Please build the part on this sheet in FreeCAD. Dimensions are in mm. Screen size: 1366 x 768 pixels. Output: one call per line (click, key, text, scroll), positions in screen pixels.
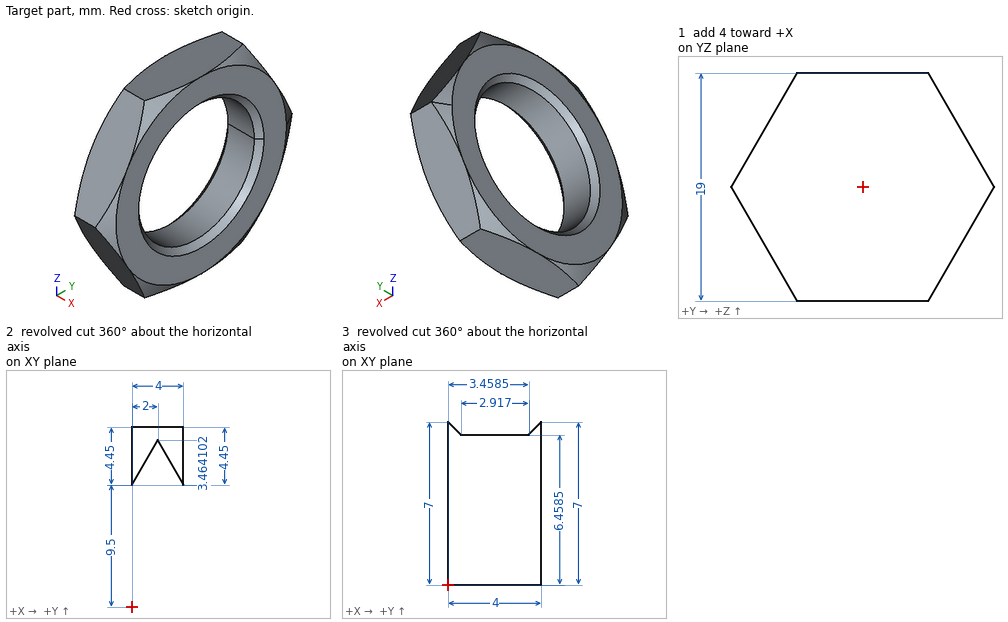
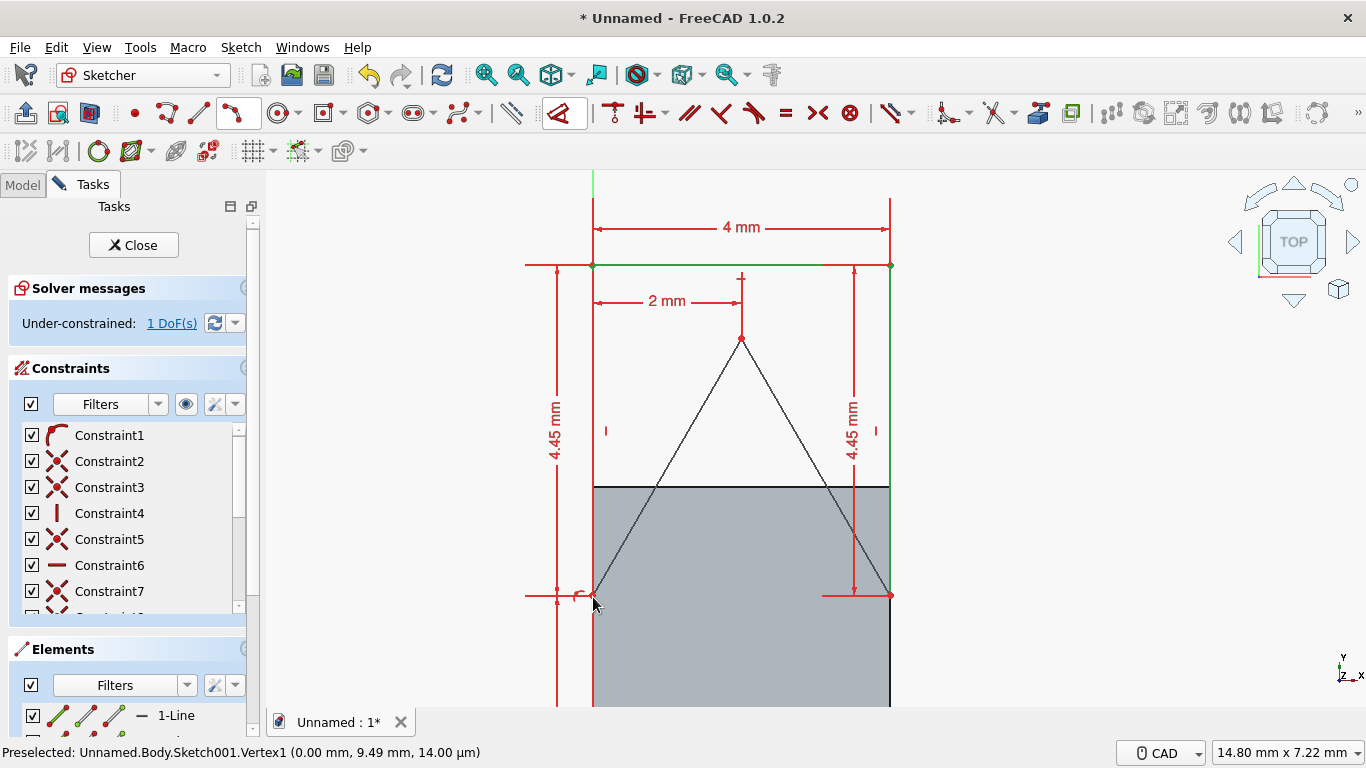
click(637, 519)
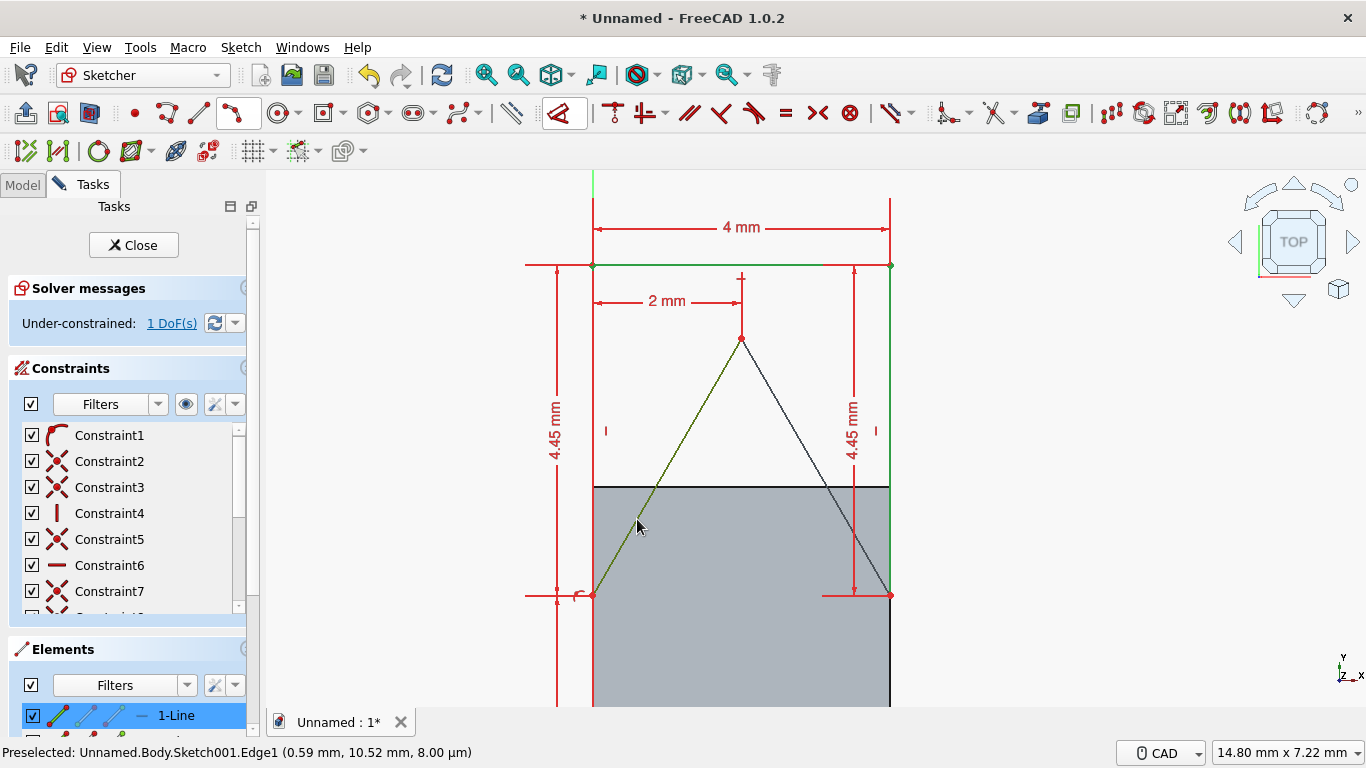
key(i)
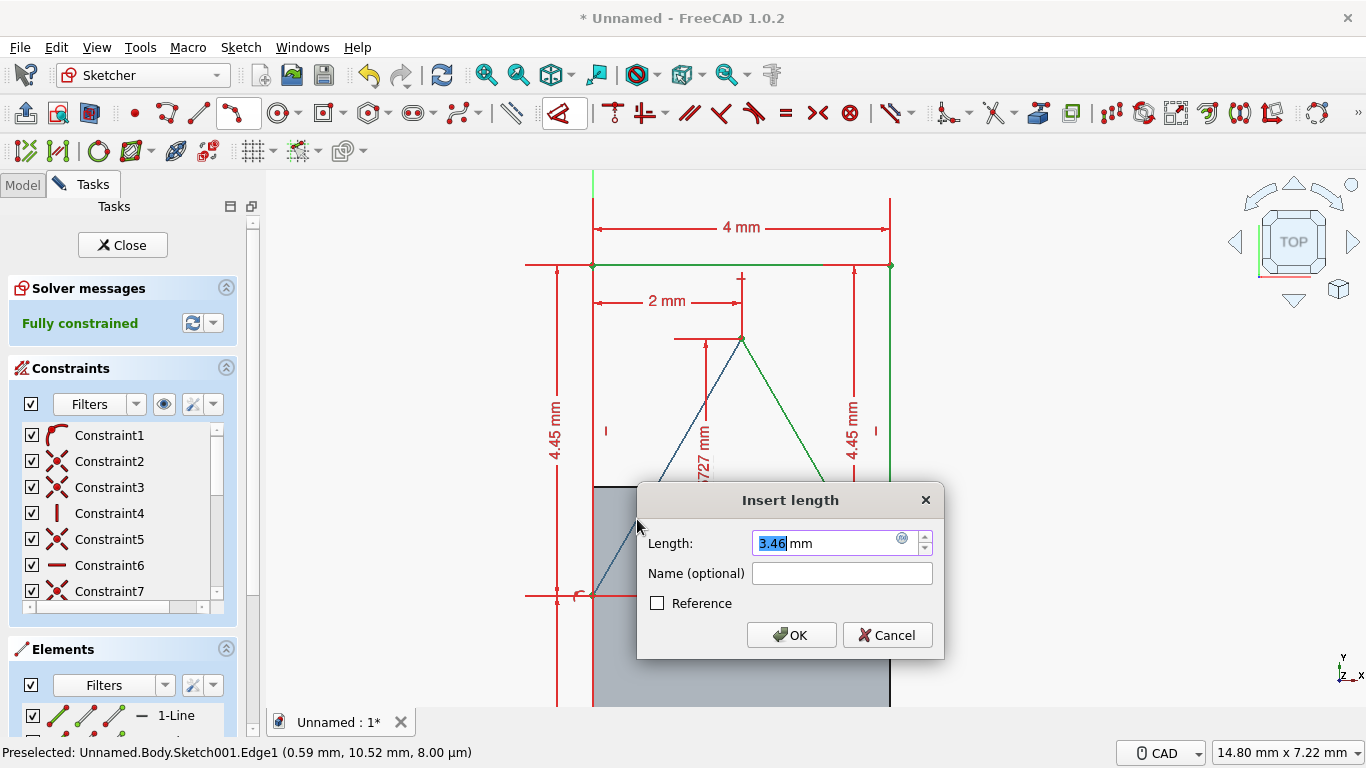
text(3.464102)
key(Return)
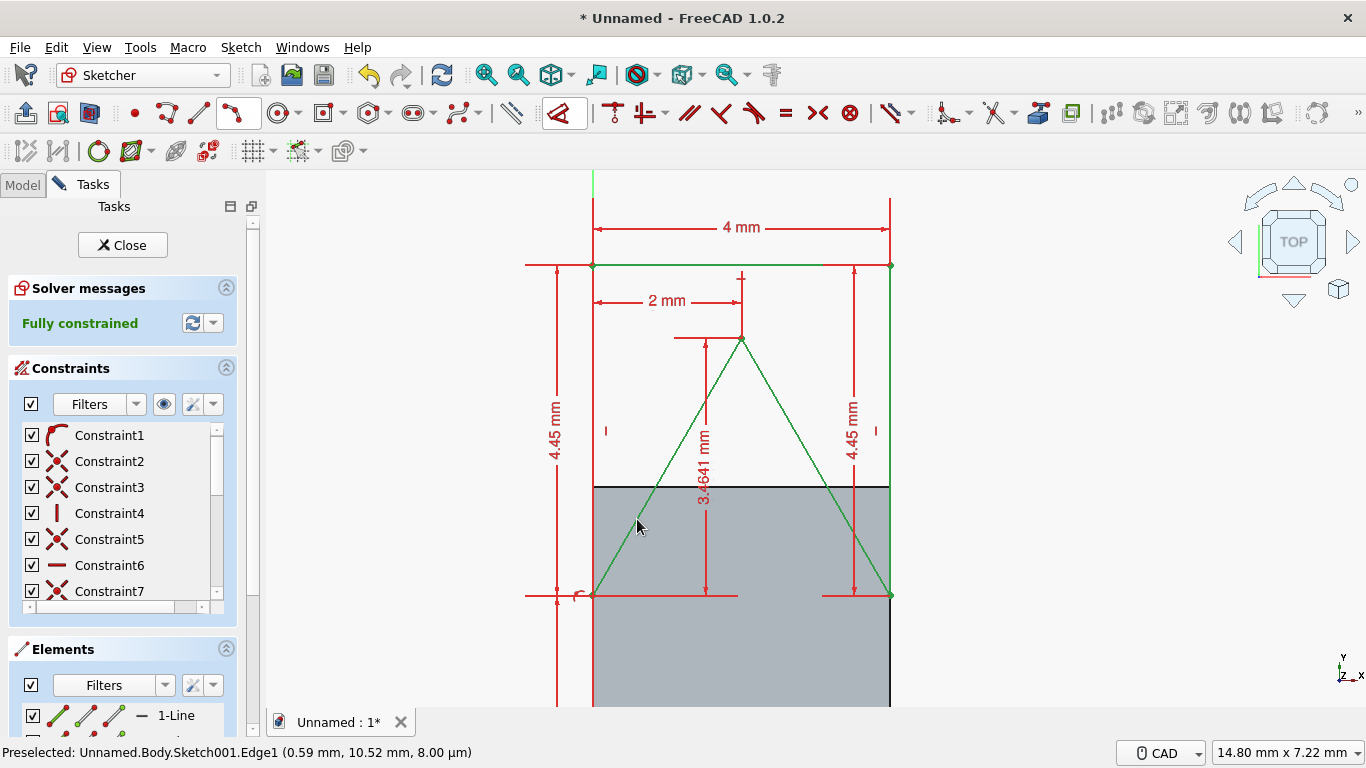
click(123, 245)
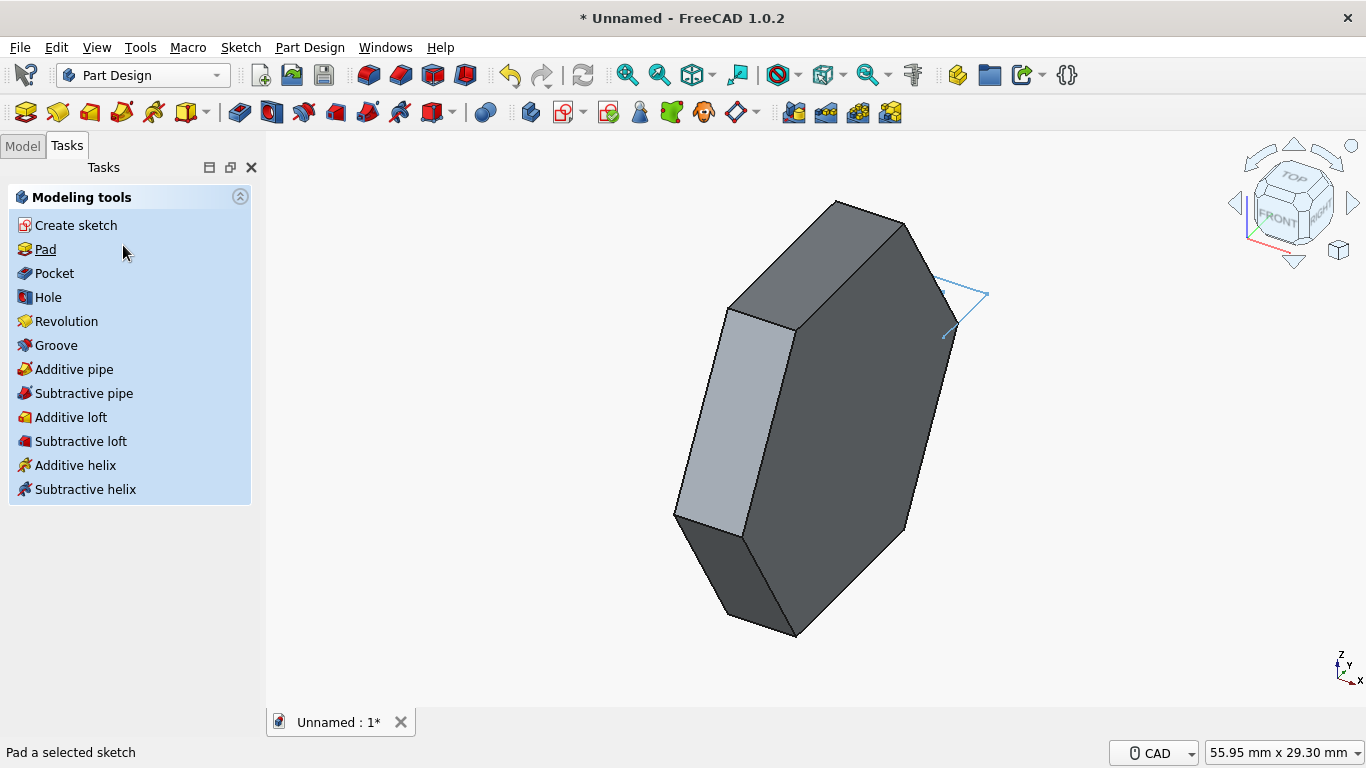
click(304, 112)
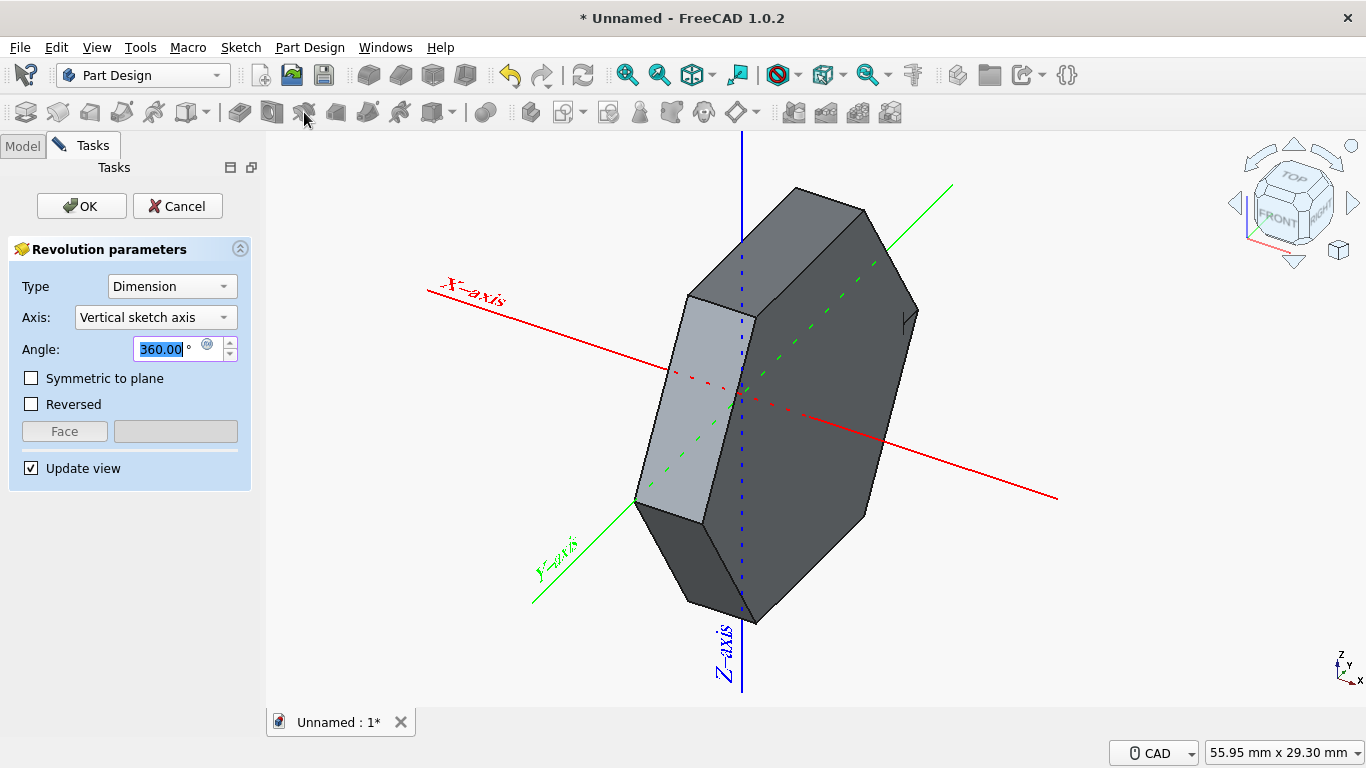
click(156, 318)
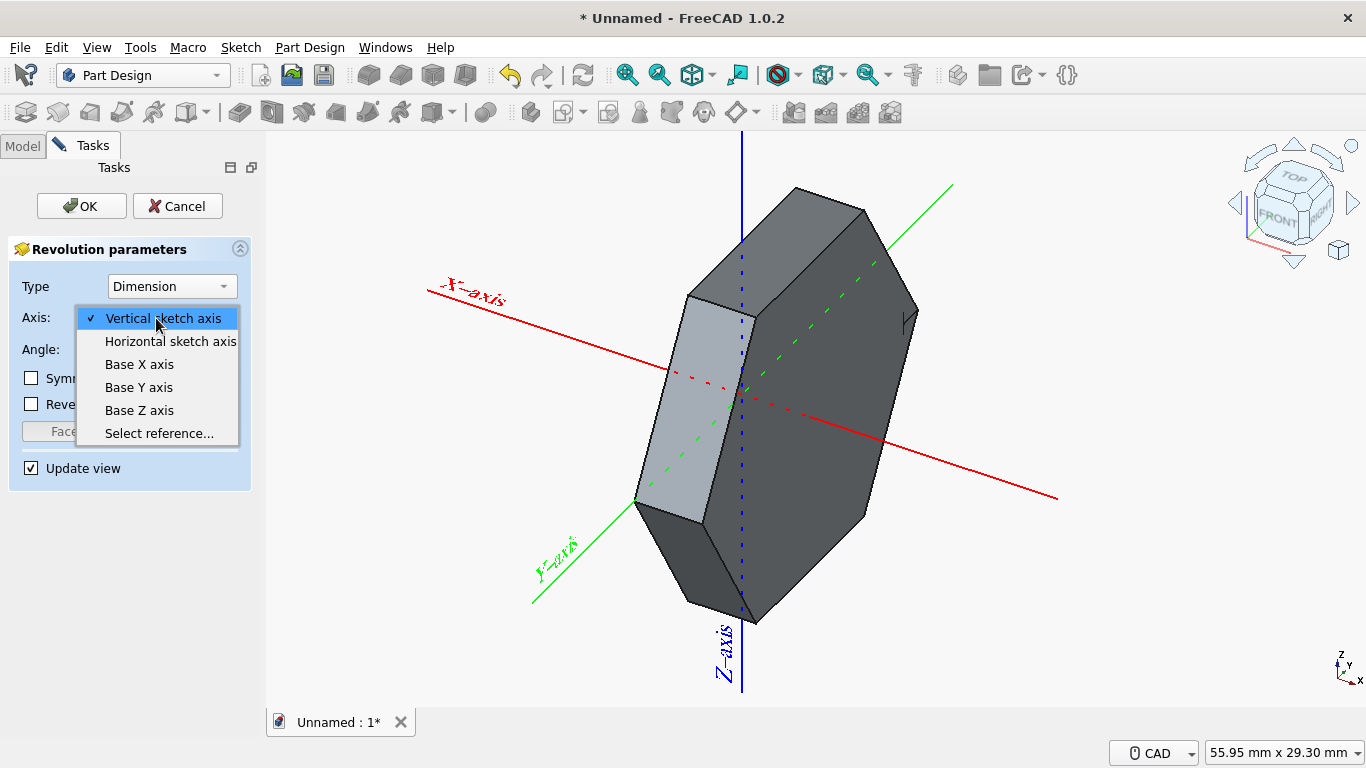
click(156, 342)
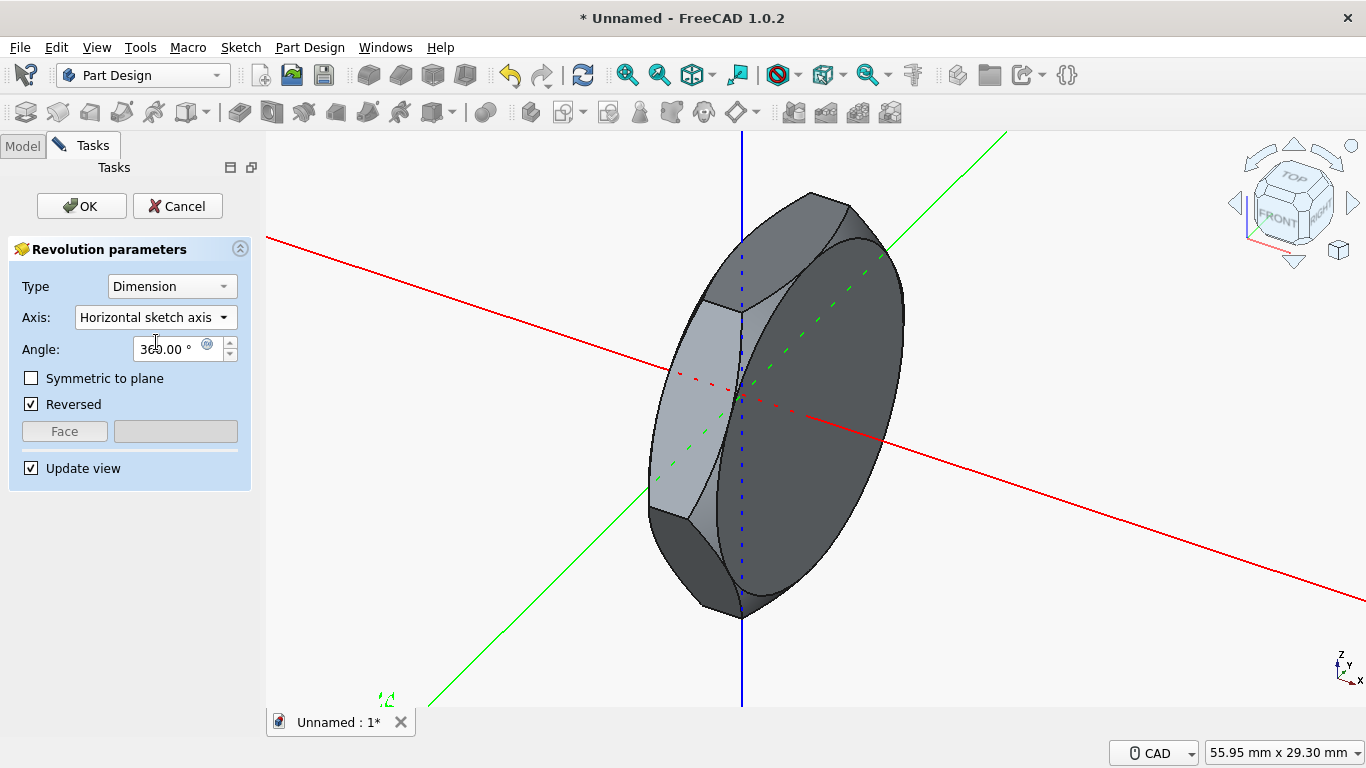
click(82, 206)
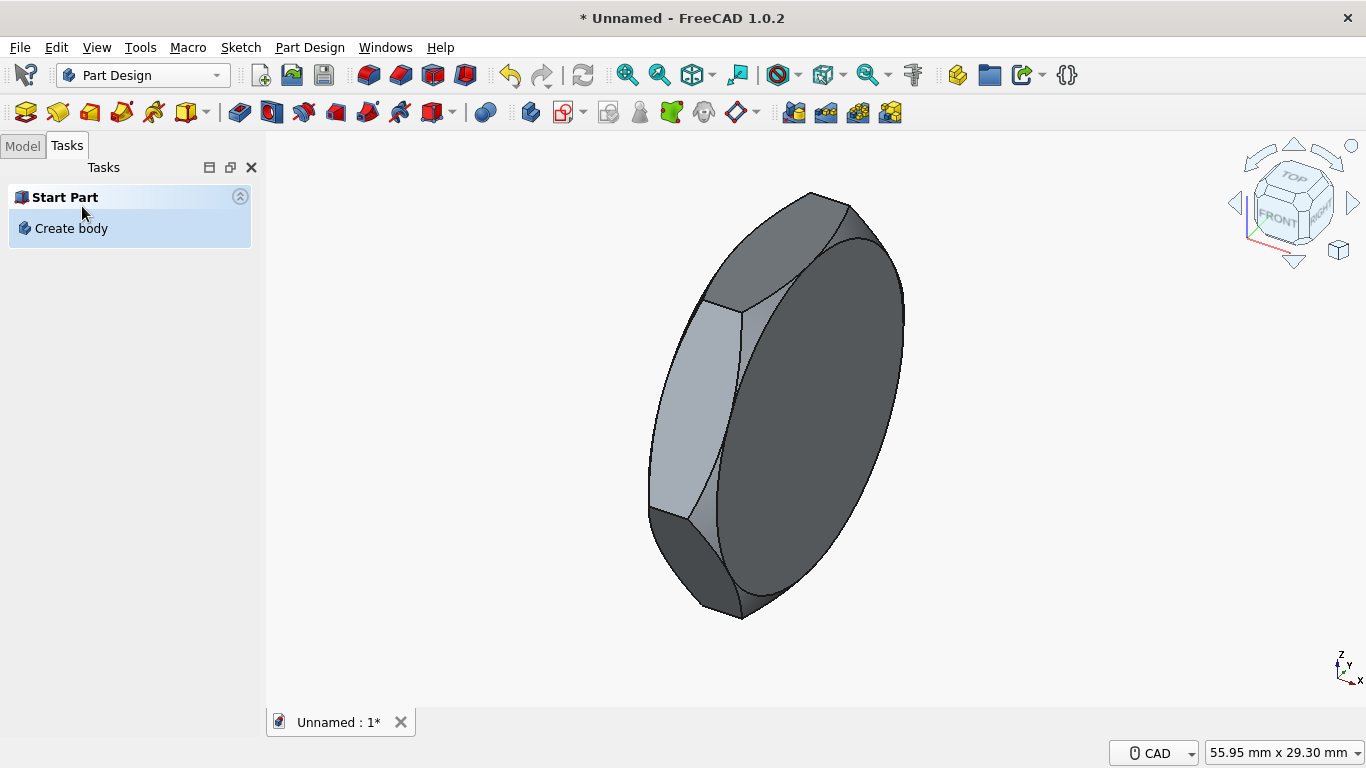
click(564, 112)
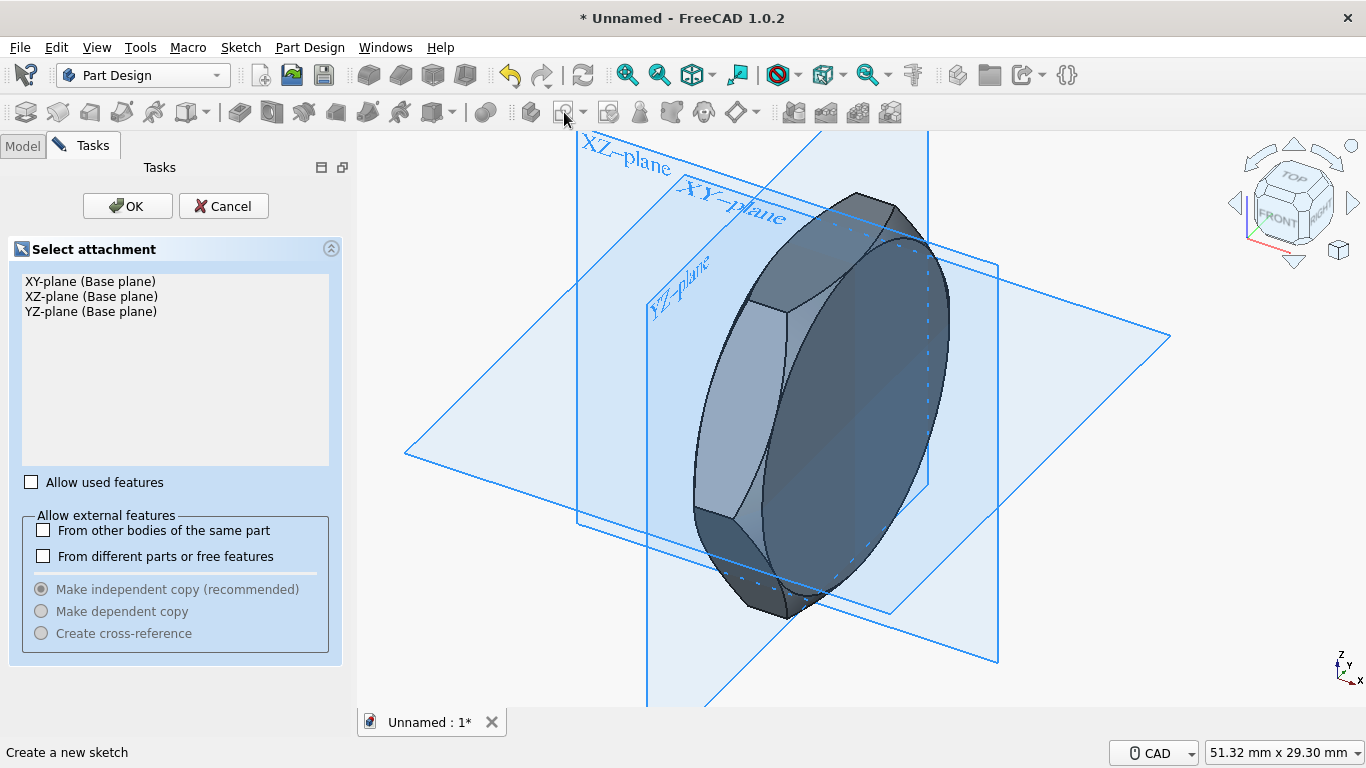
click(82, 282)